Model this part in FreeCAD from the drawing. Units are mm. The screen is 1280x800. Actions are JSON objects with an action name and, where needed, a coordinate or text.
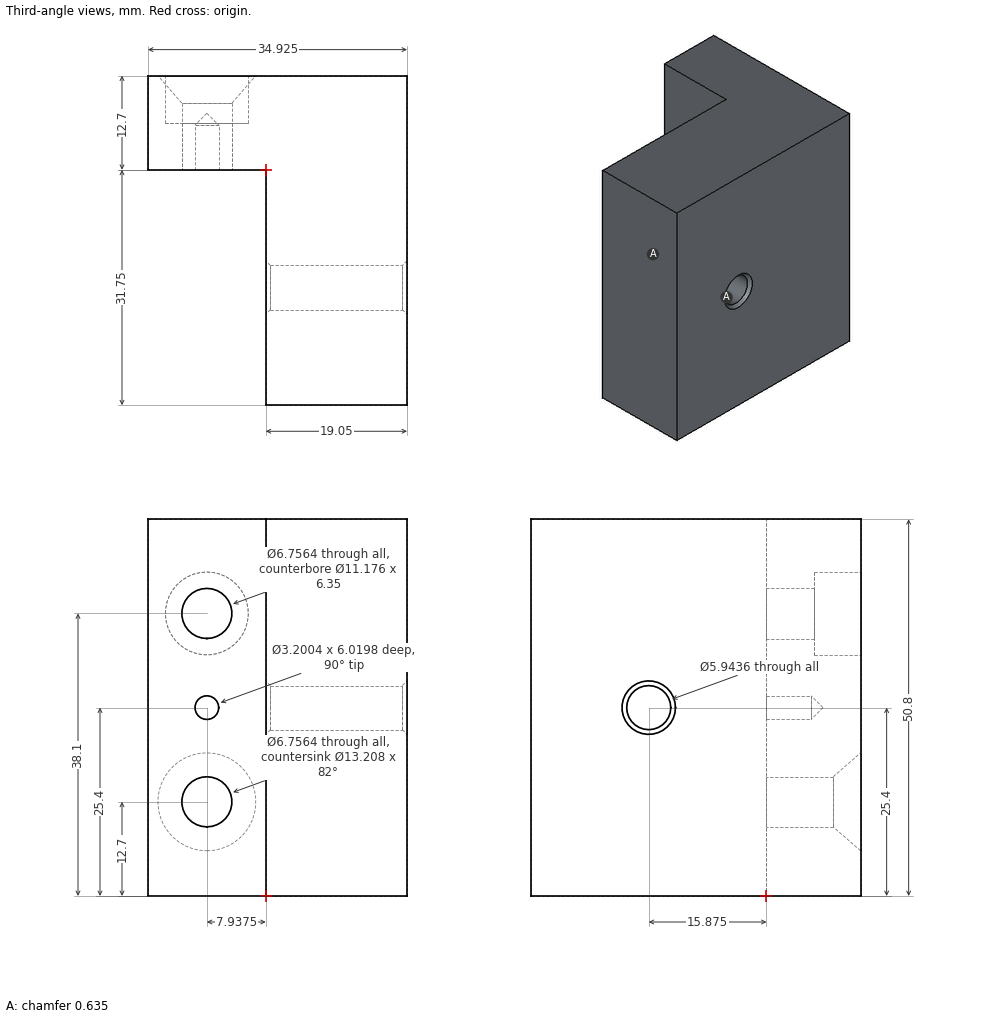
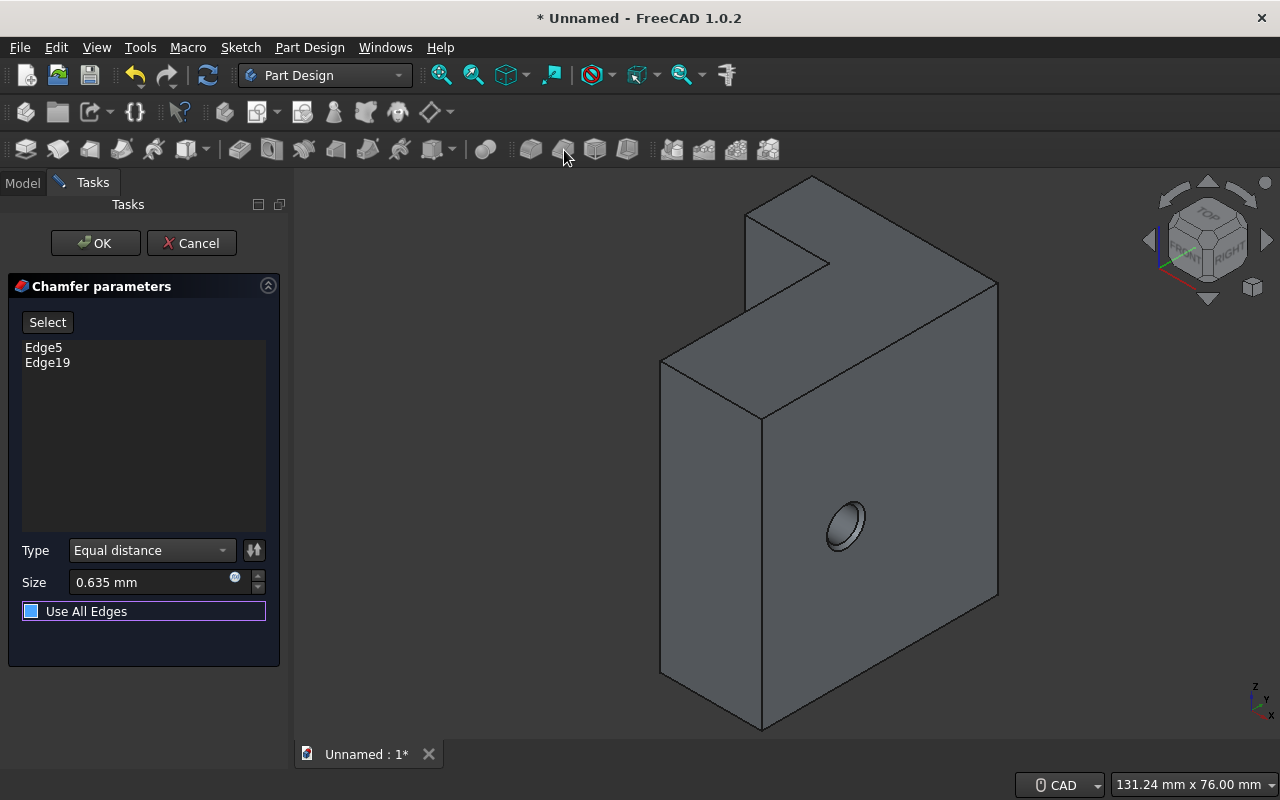
{"action": "left_click", "coordinate": [96, 243]}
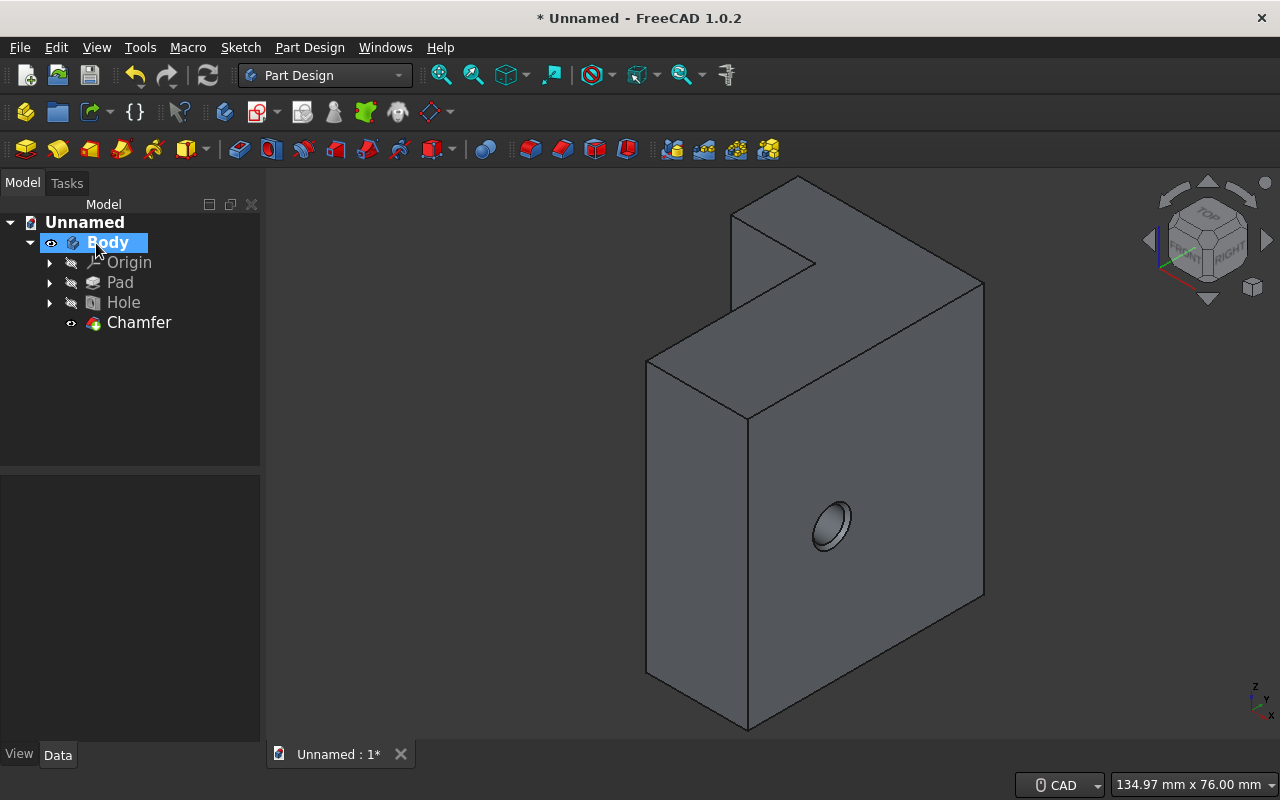
{"action": "left_click", "coordinate": [258, 112]}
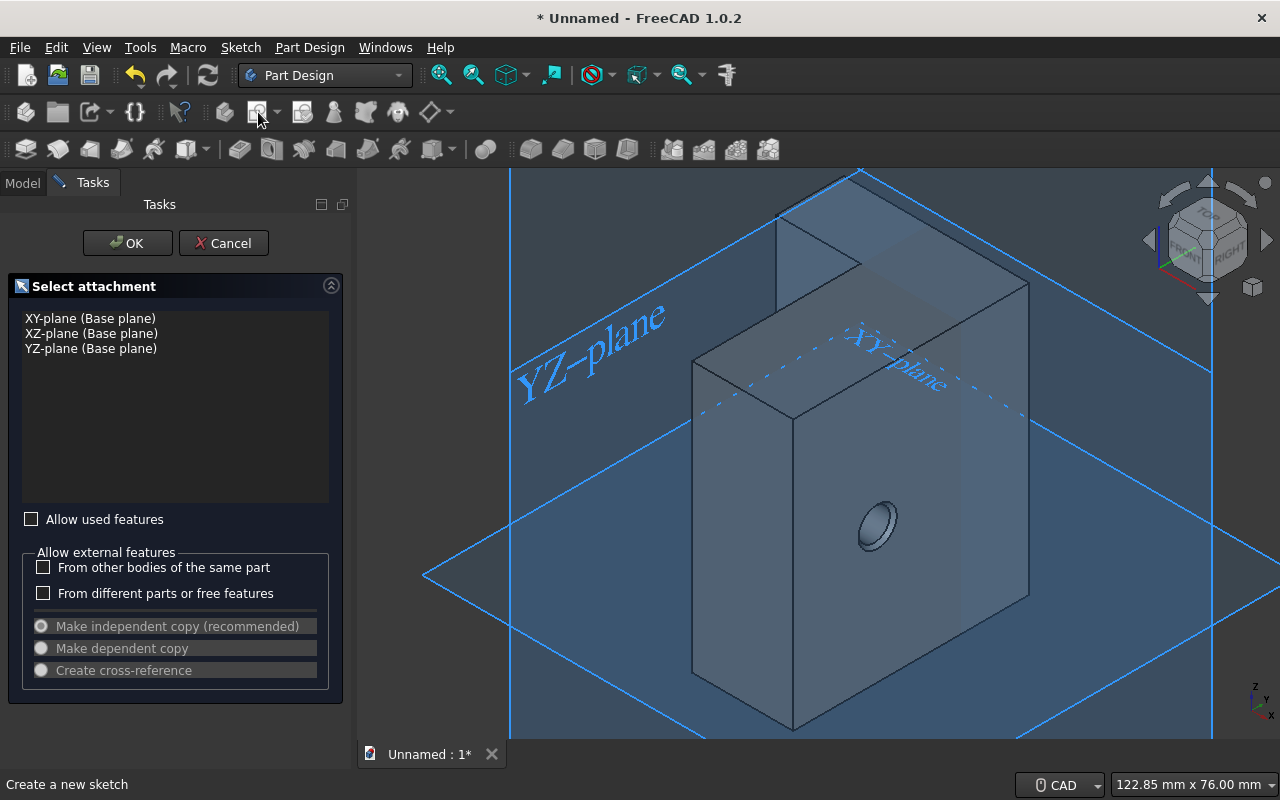
{"action": "left_click", "coordinate": [82, 334]}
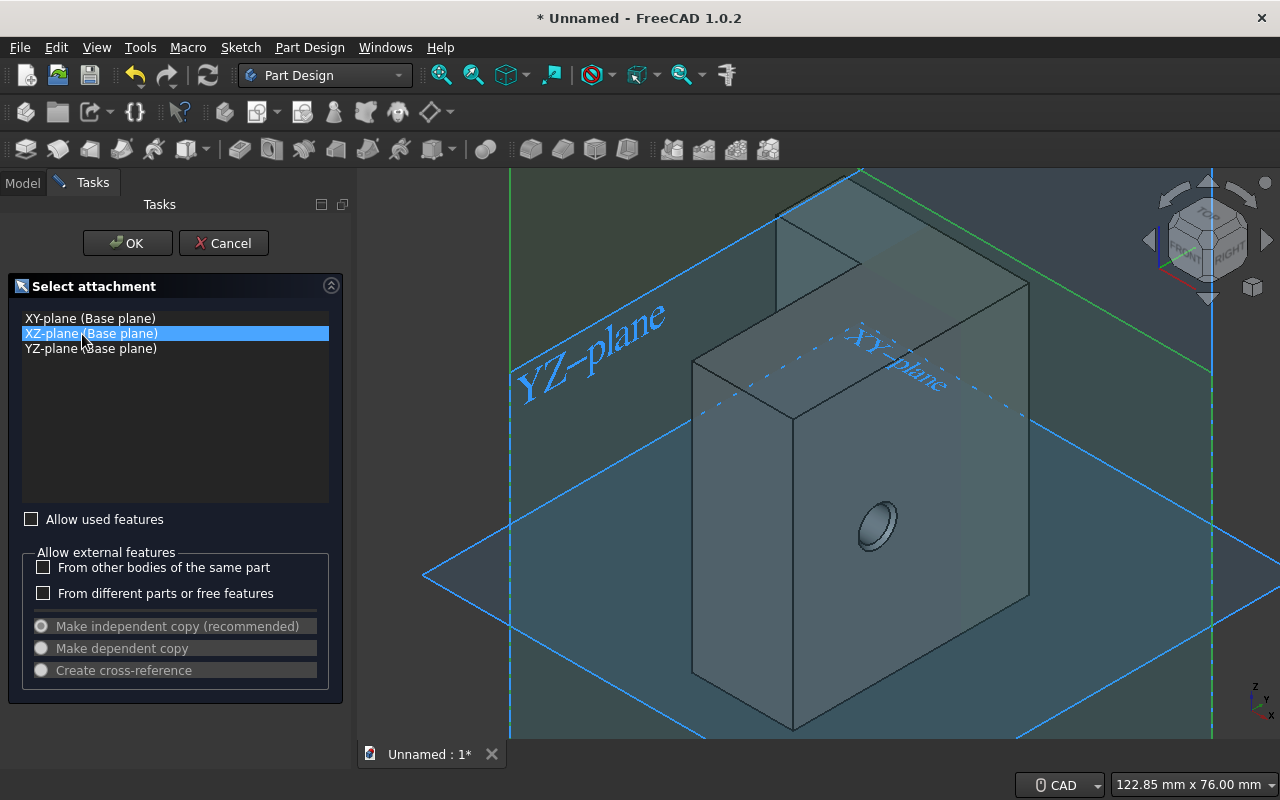
{"action": "left_click", "coordinate": [128, 243]}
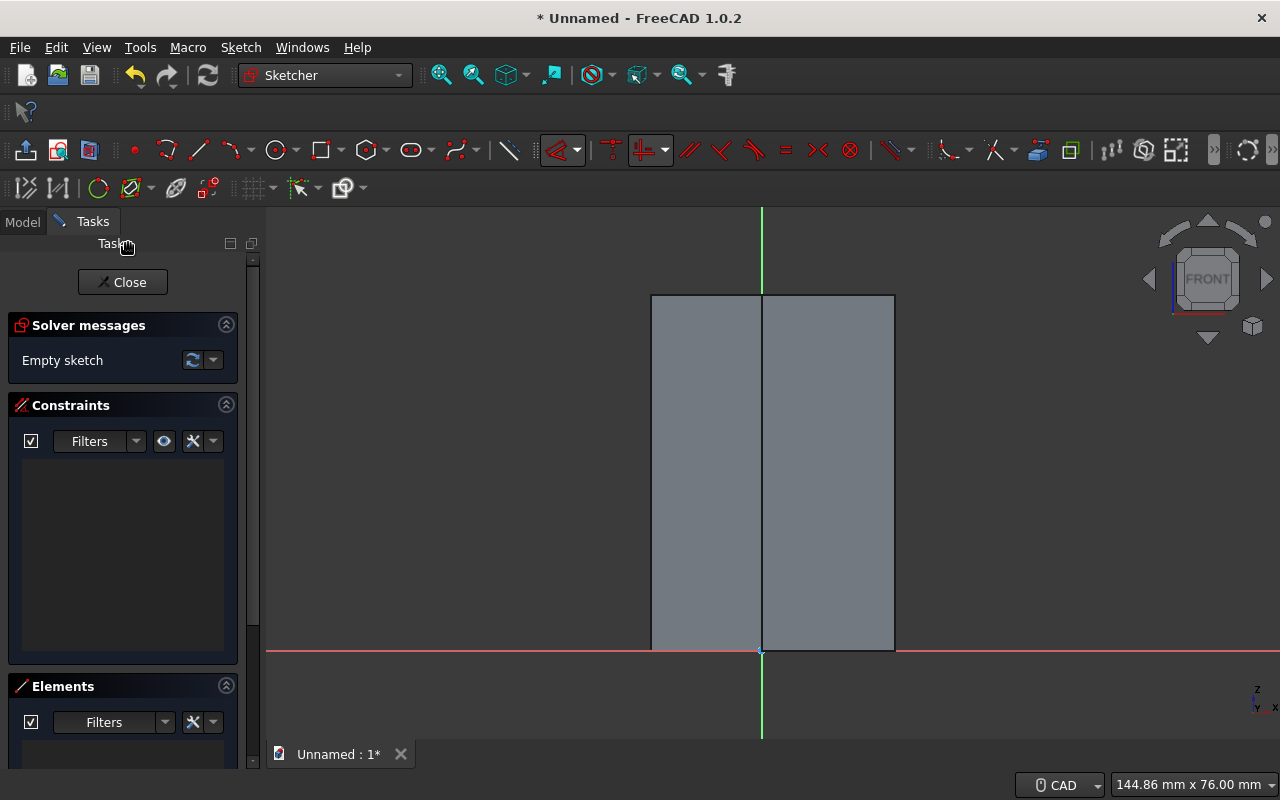
{"action": "left_click", "coordinate": [90, 150]}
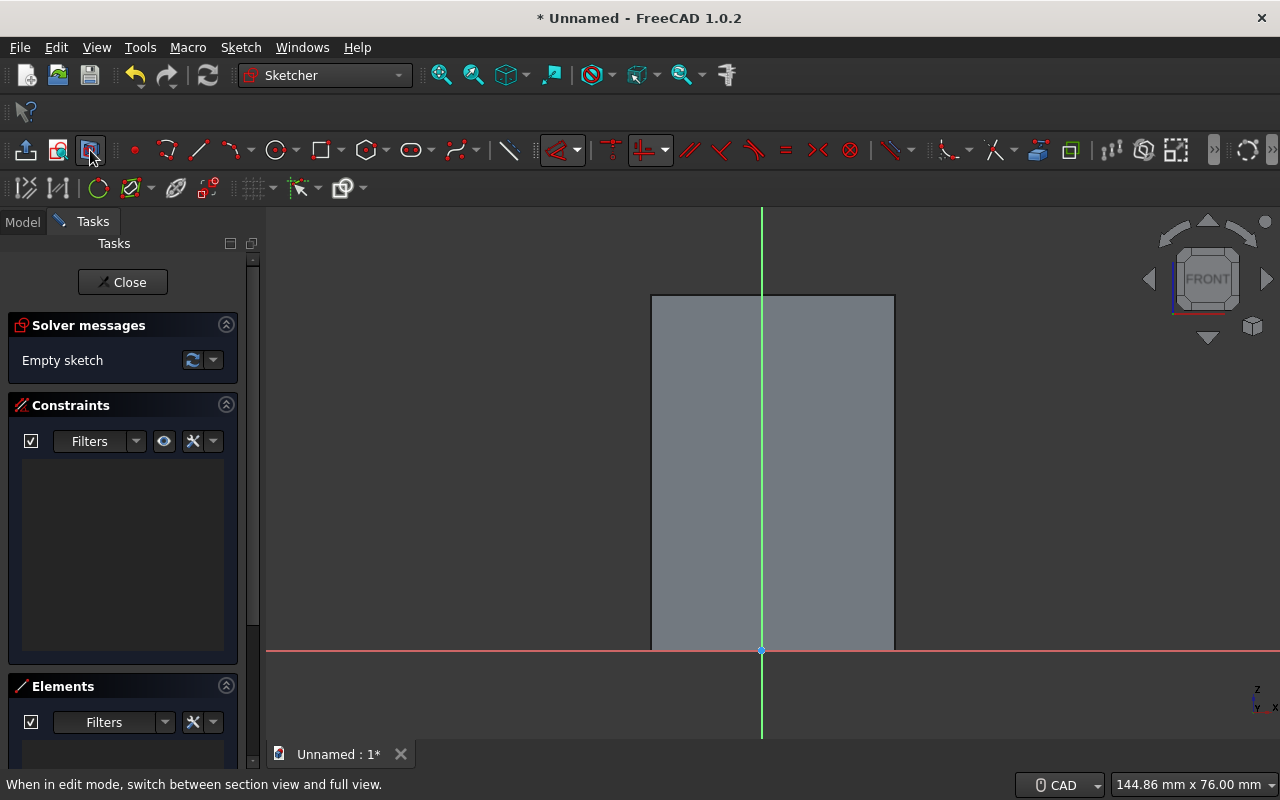
{"action": "scroll", "coordinate": [706, 473], "scroll_direction": "up", "scroll_amount": 14}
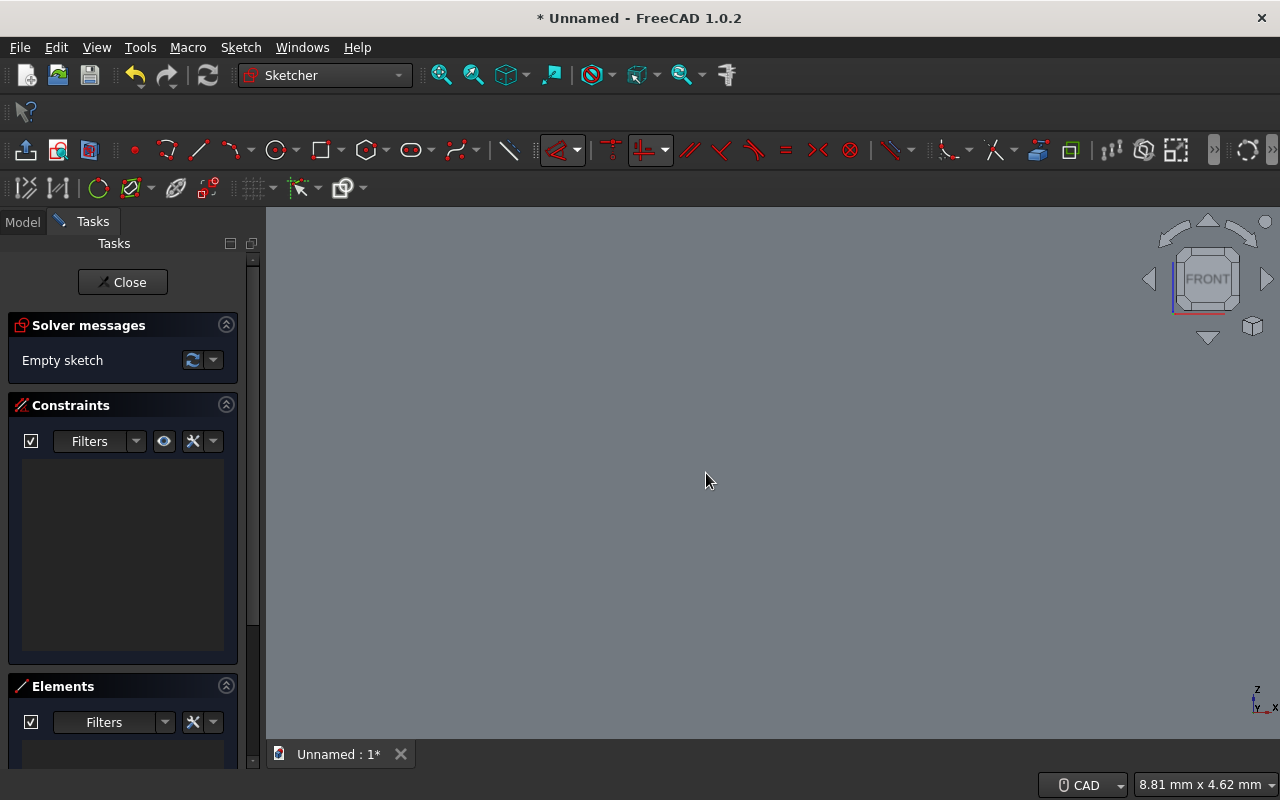
{"action": "left_click", "coordinate": [276, 150]}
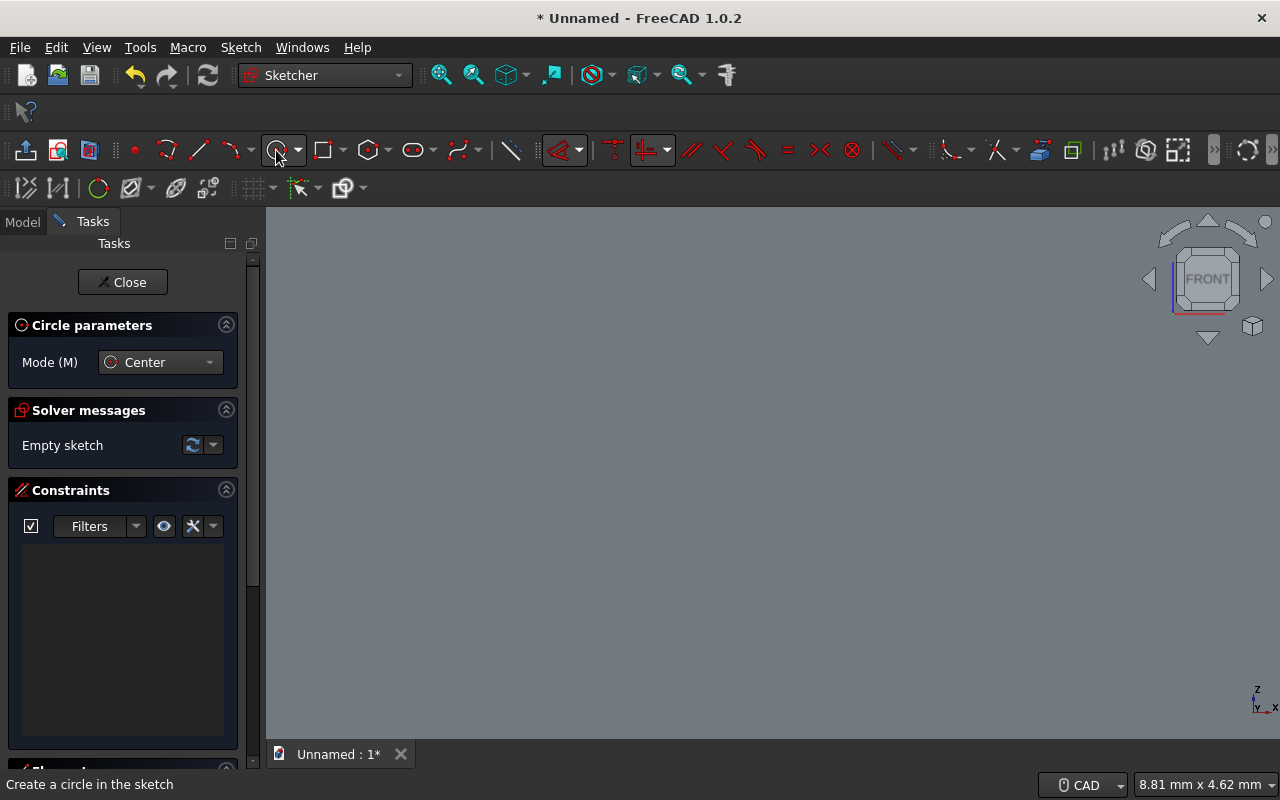
{"action": "left_click", "coordinate": [705, 465]}
{"action": "mouse_move", "coordinate": [835, 335]}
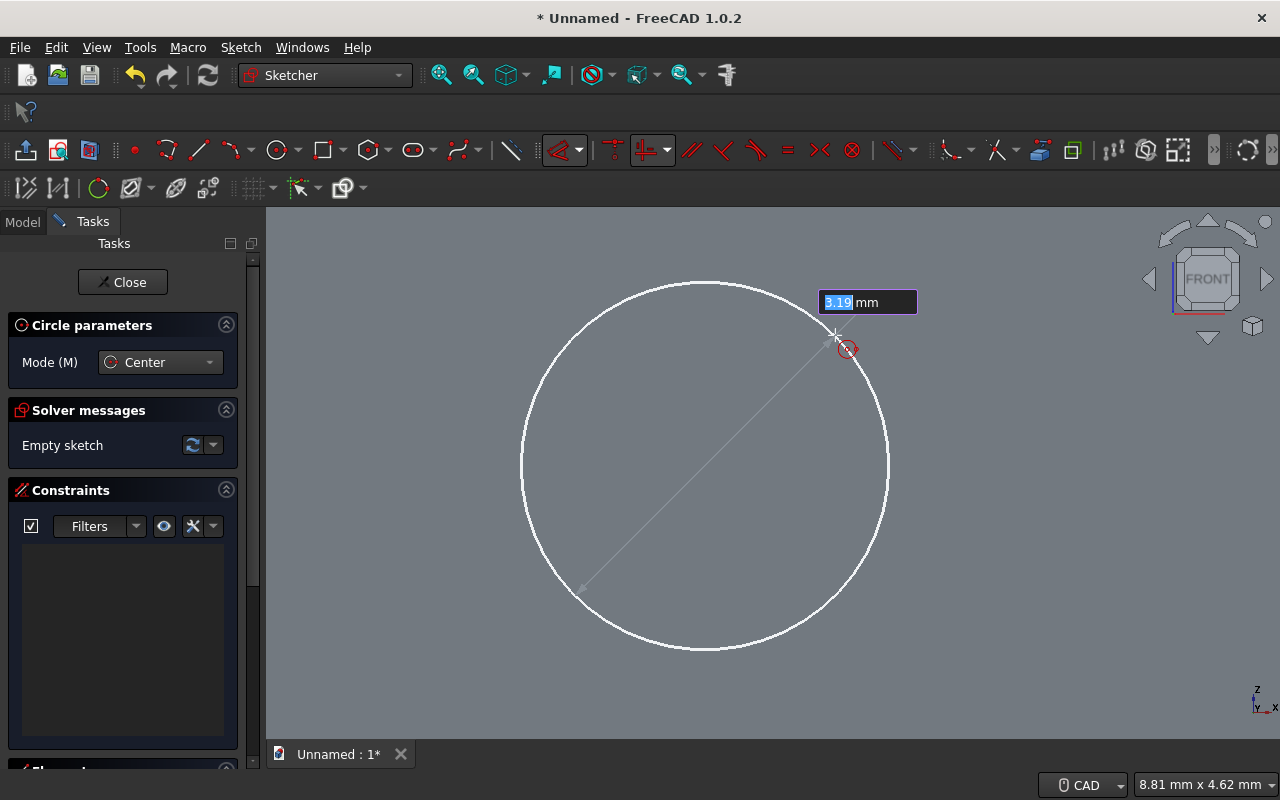
{"action": "type", "text": "3.2004"}
{"action": "key", "text": "Return"}
{"action": "key", "text": "Escape"}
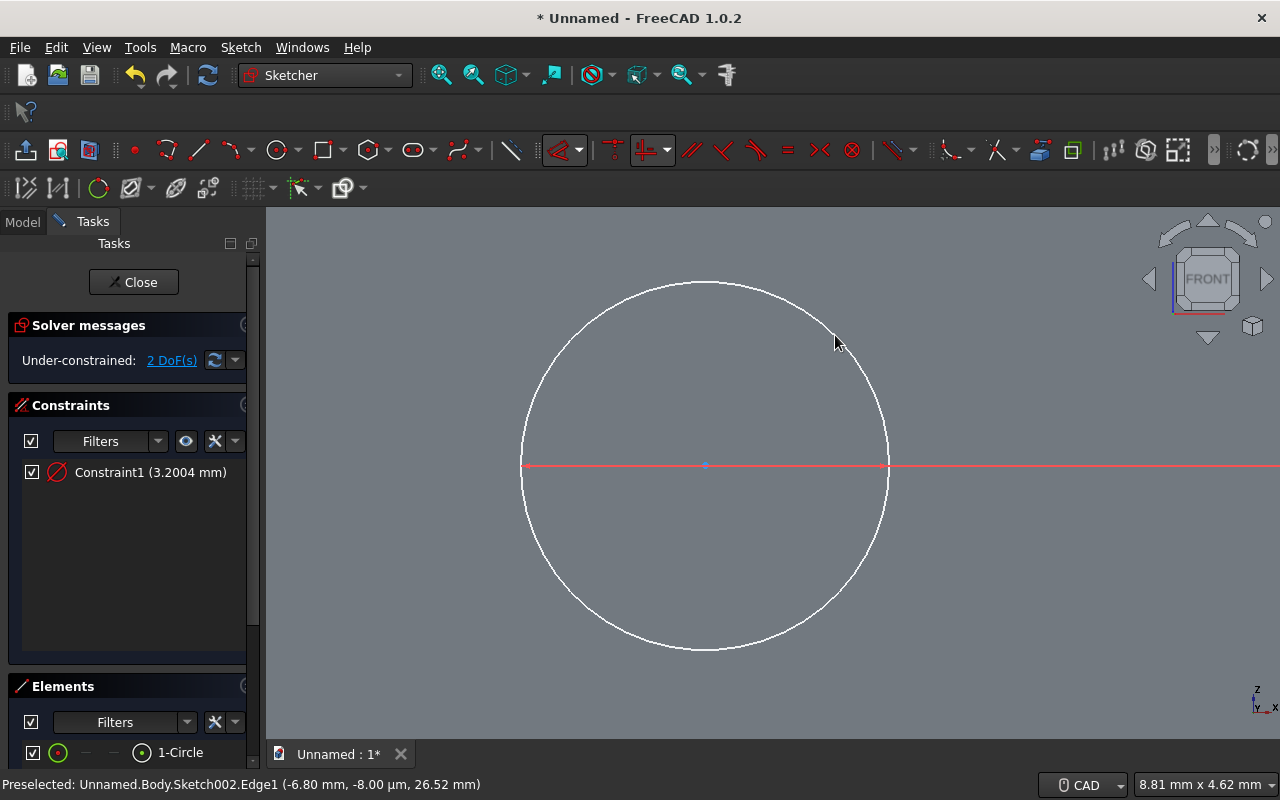
{"action": "left_click", "coordinate": [705, 466]}